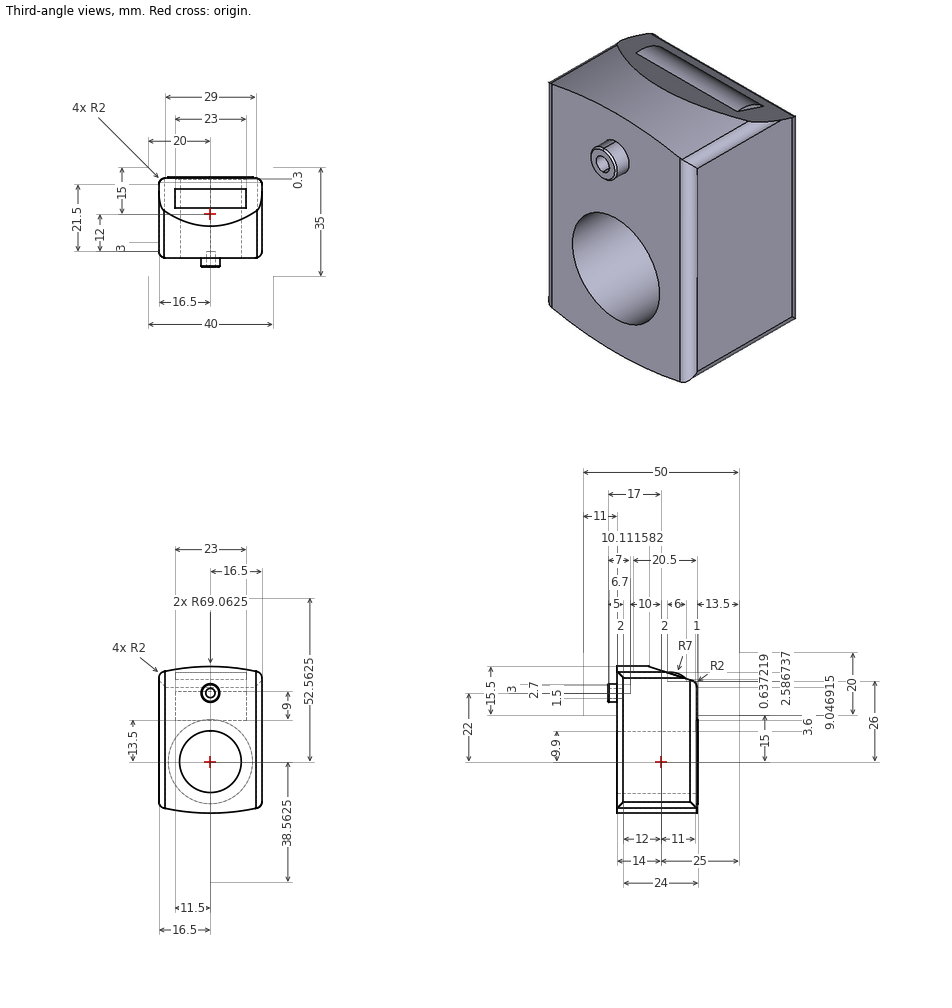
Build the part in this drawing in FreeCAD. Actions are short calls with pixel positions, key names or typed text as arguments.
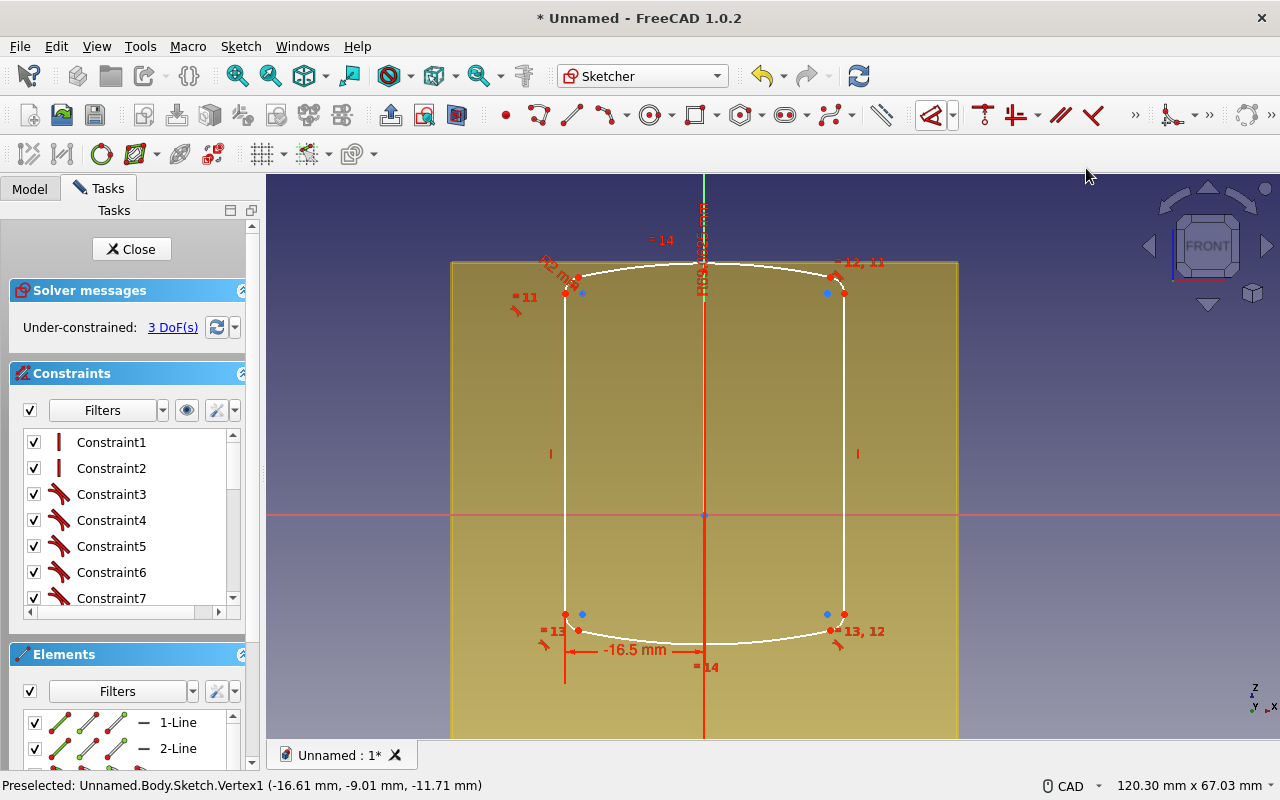
click(844, 294)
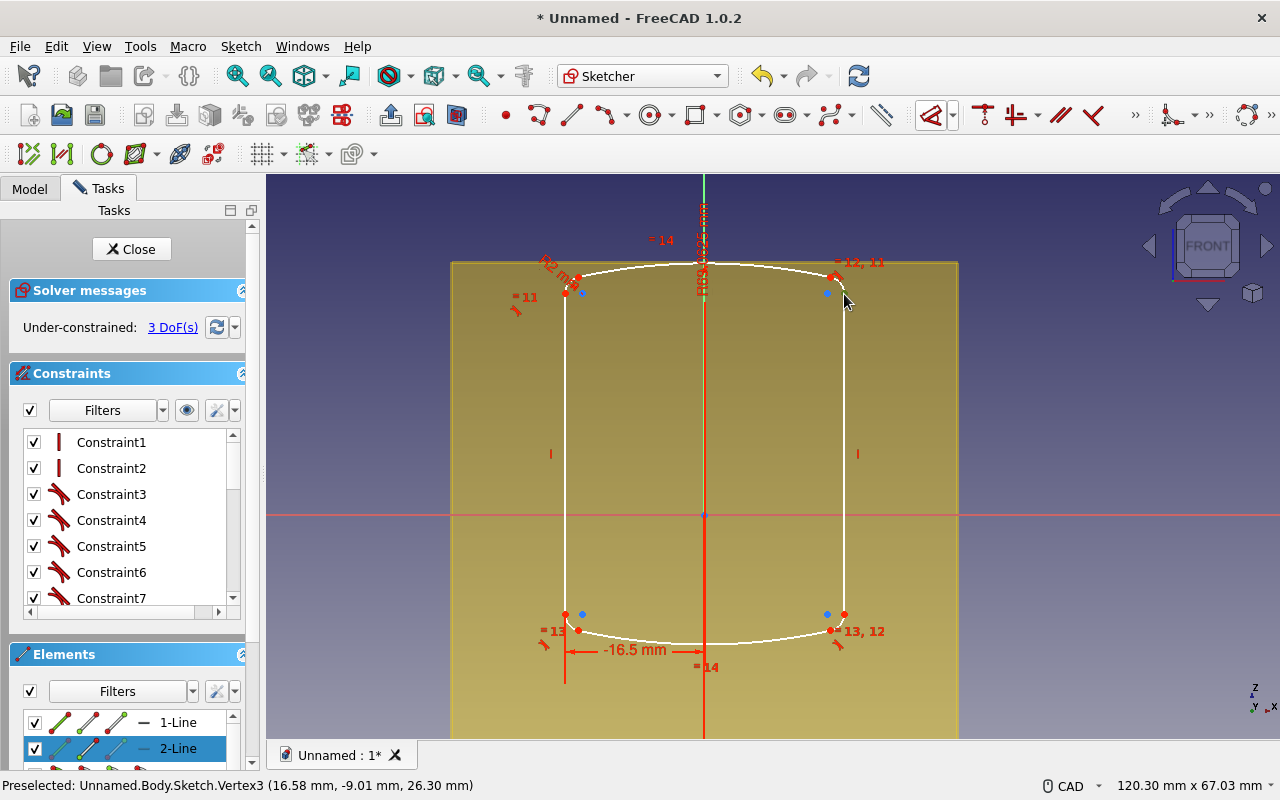
key(l)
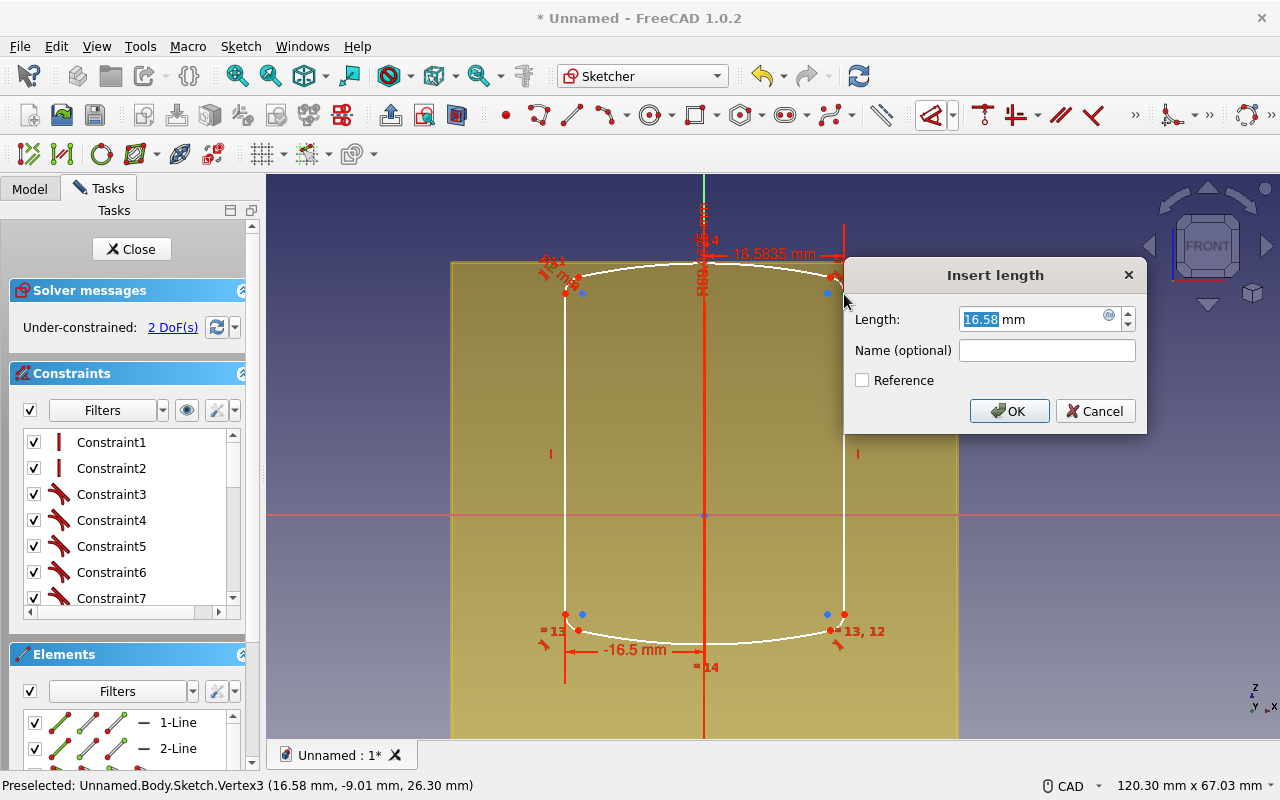
text(16.5)
key(Return)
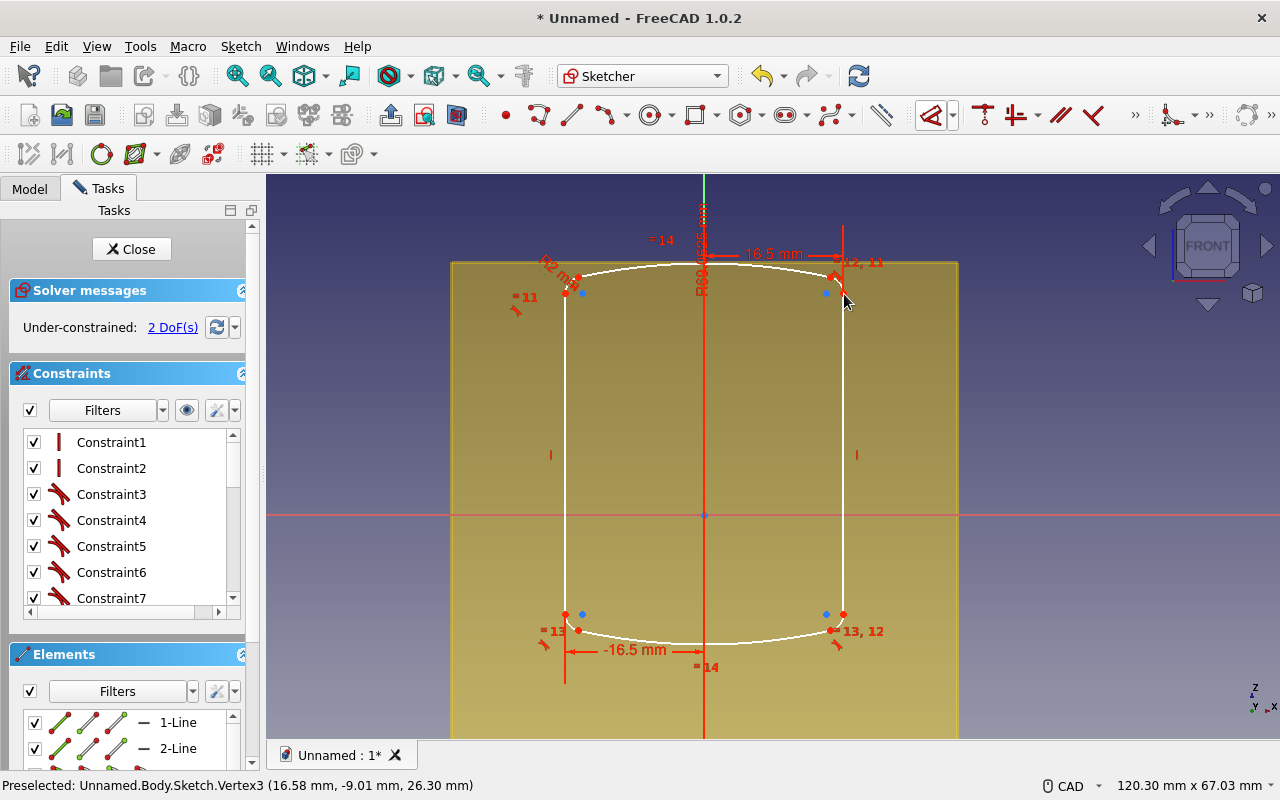
scroll(705, 262, down, 2)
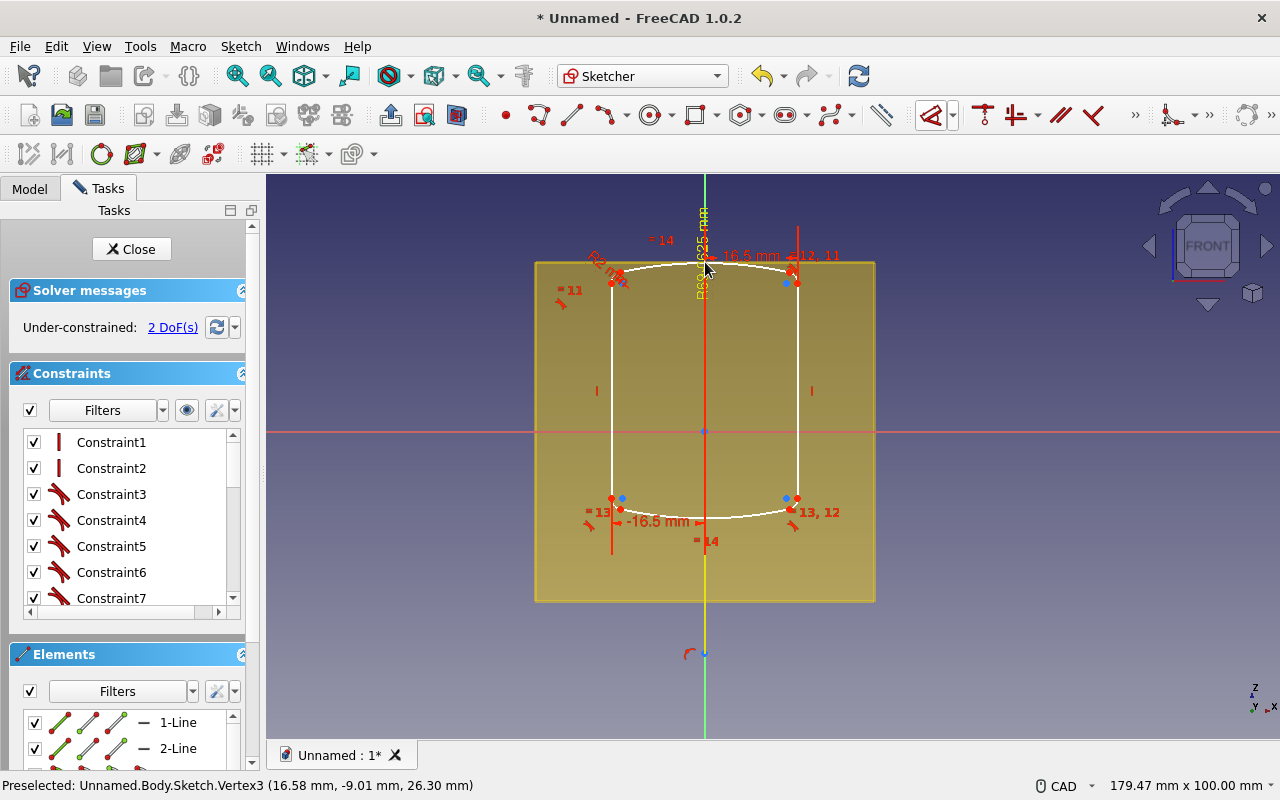
click(705, 653)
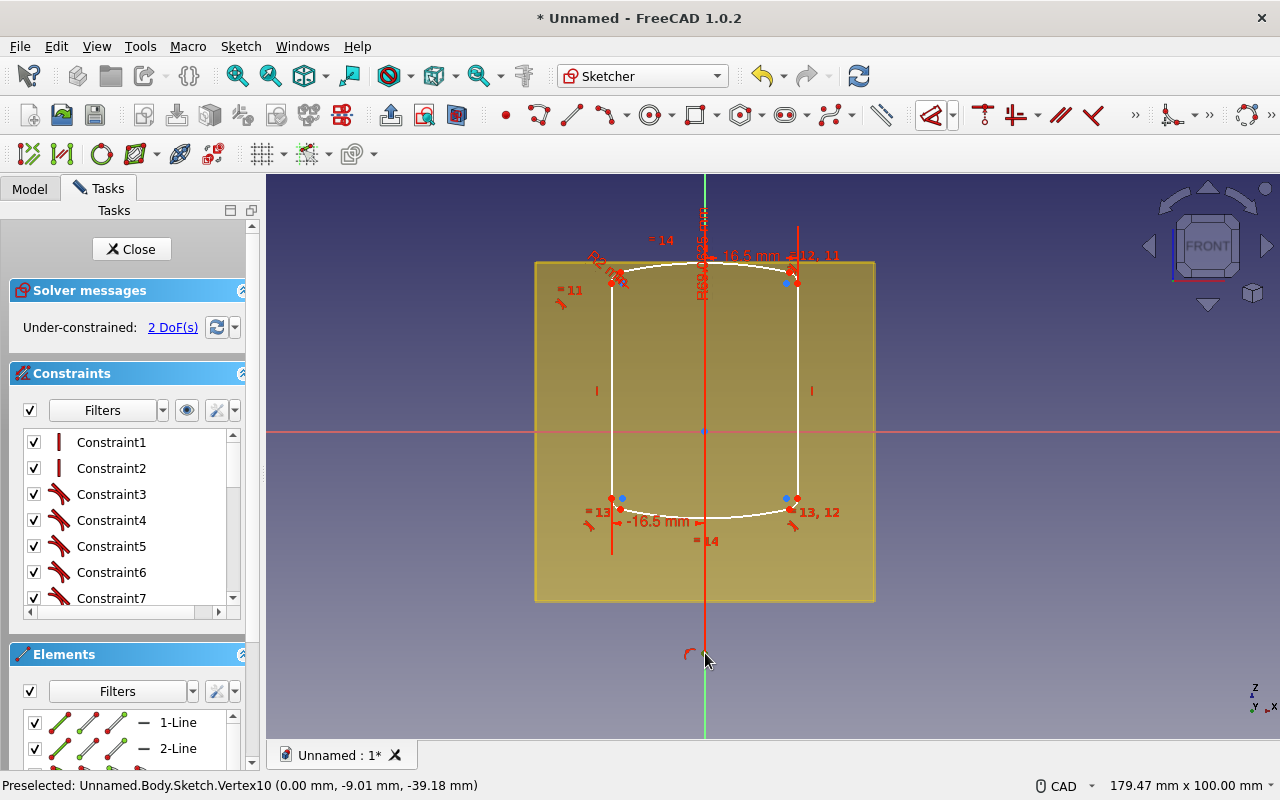
click(952, 116)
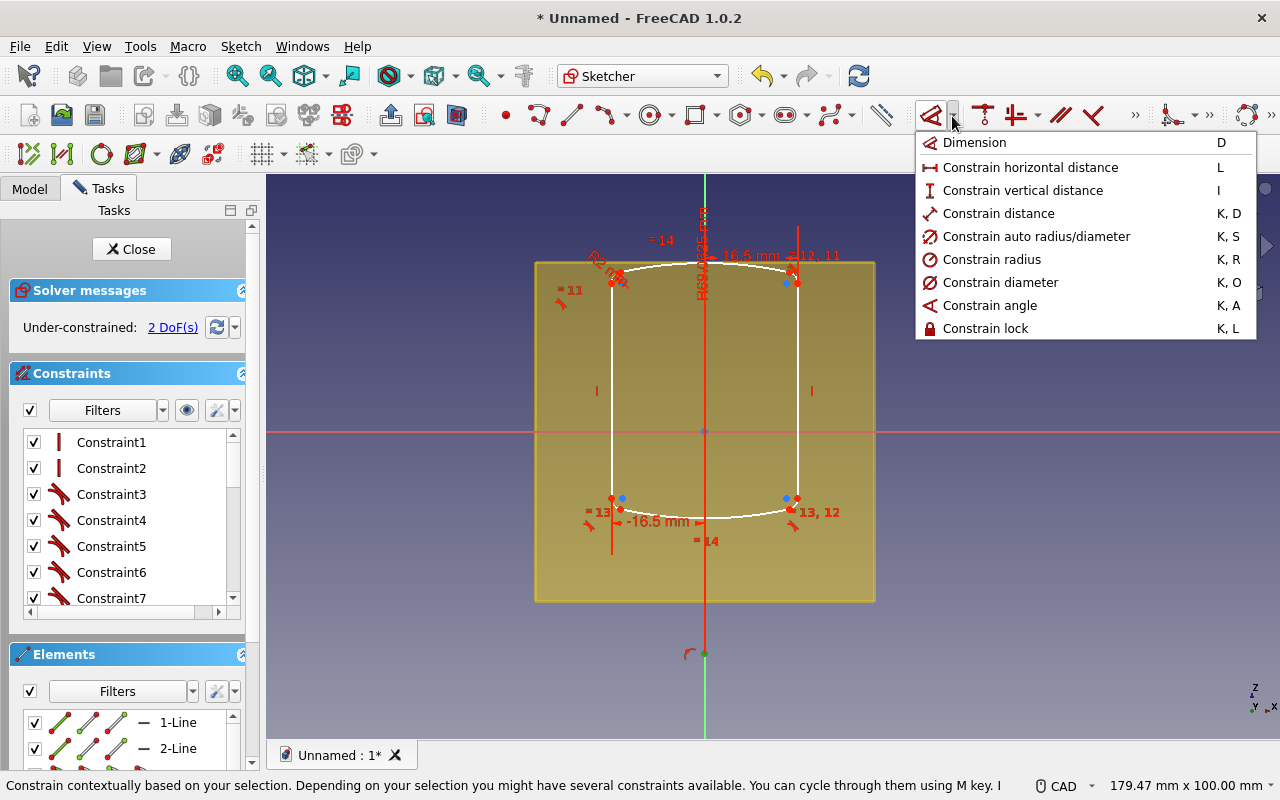
click(1086, 190)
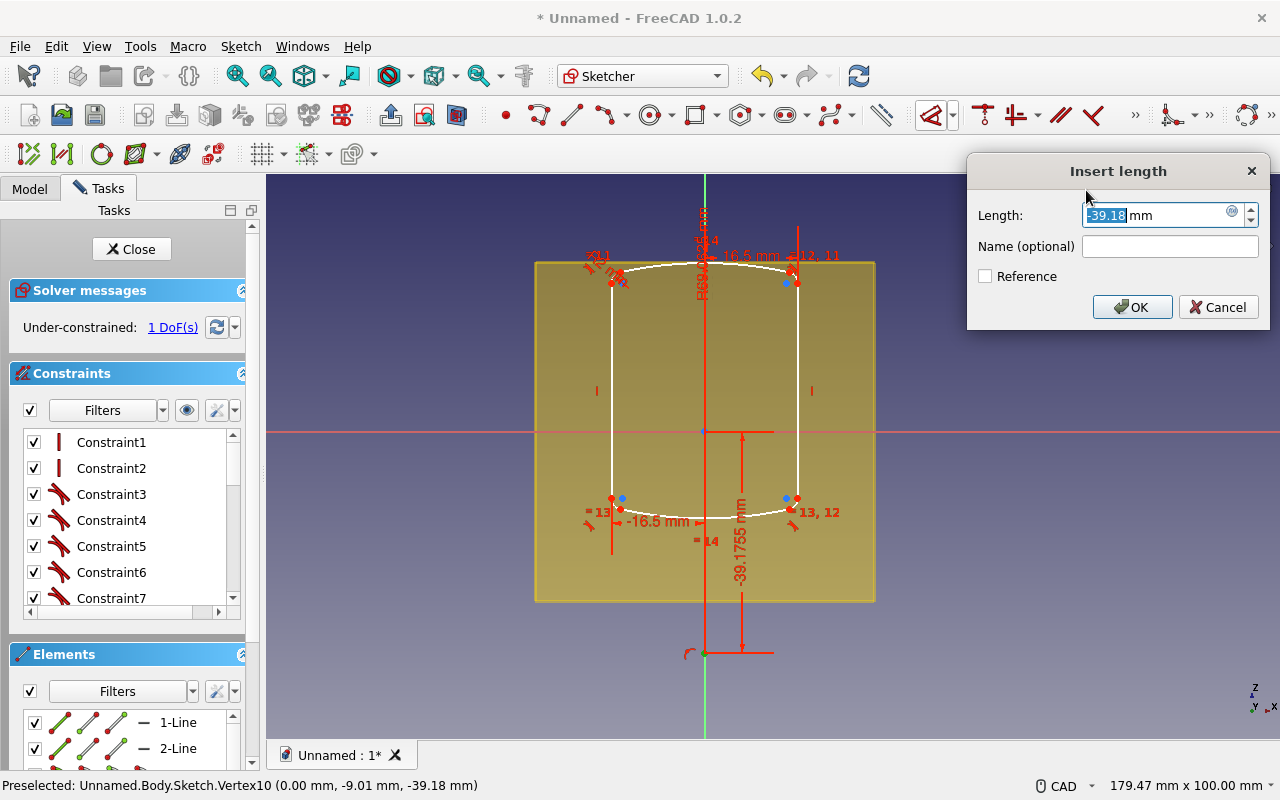
text(-38.5625)
key(Return)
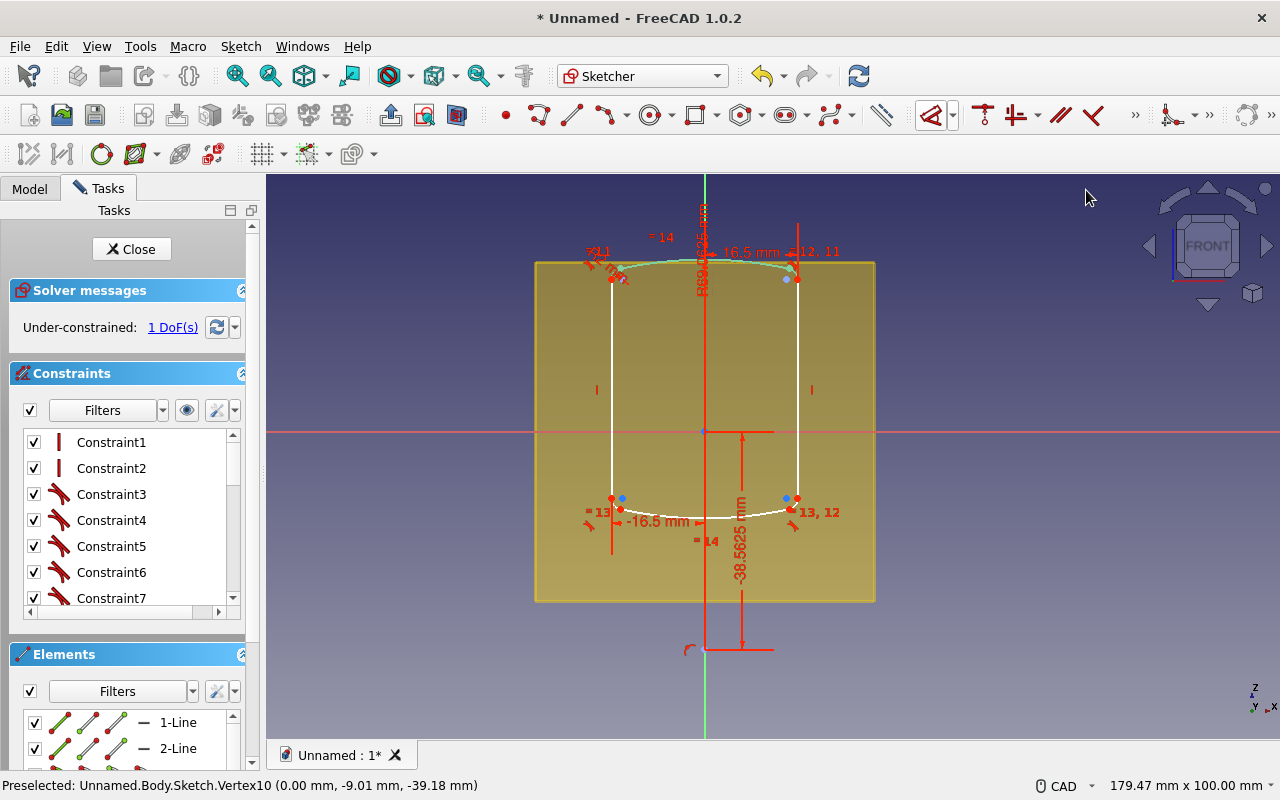
scroll(705, 262, up, 2)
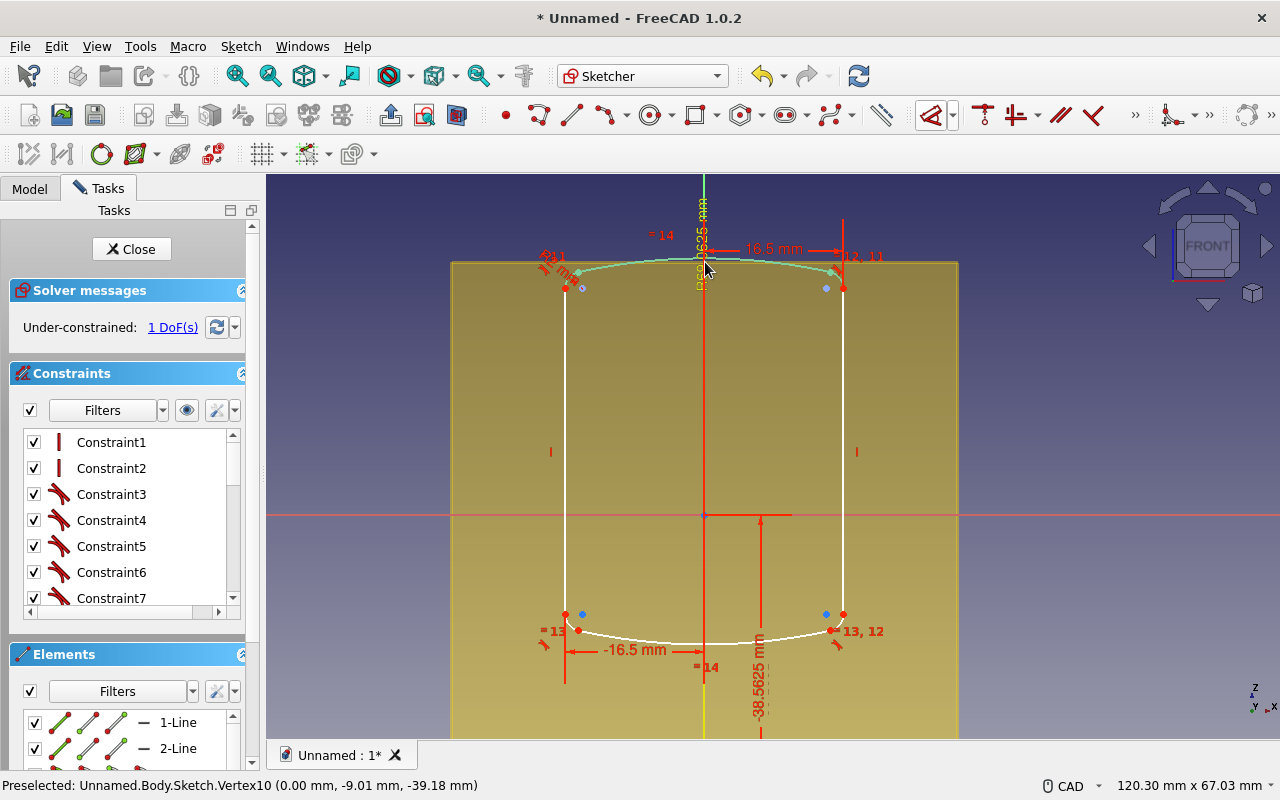
scroll(705, 656, down, 2)